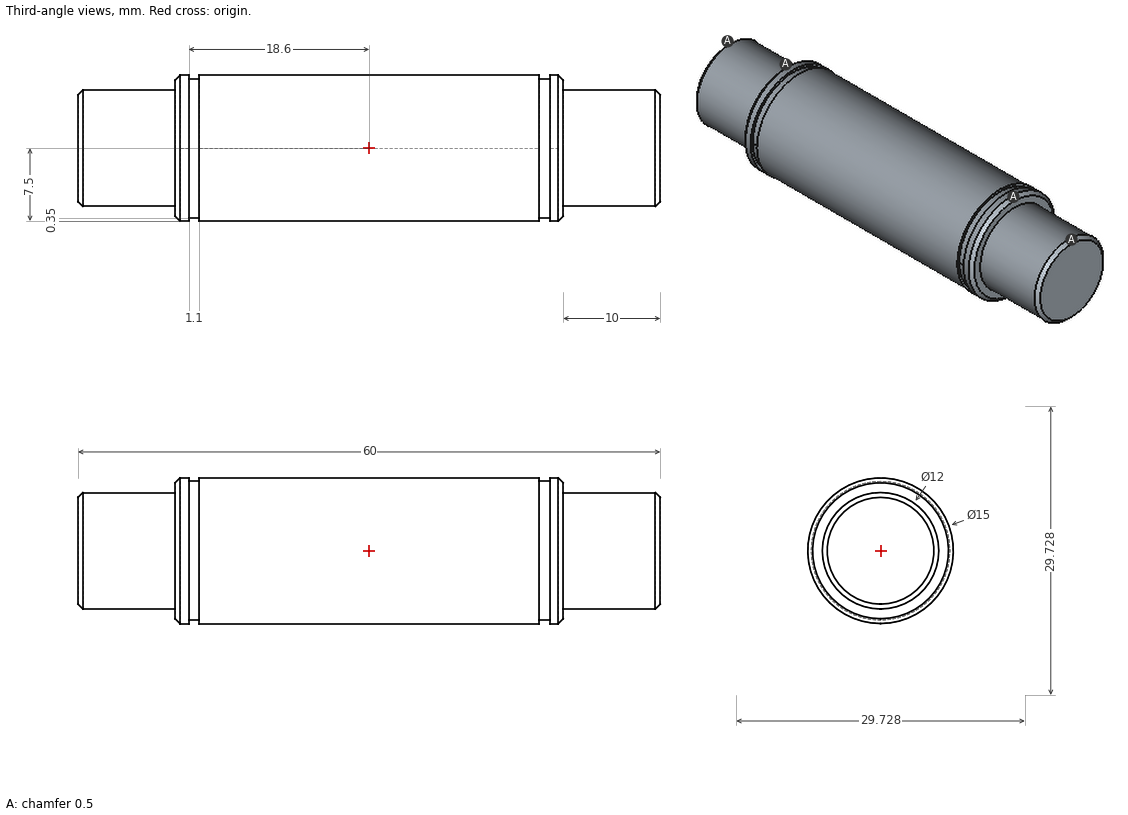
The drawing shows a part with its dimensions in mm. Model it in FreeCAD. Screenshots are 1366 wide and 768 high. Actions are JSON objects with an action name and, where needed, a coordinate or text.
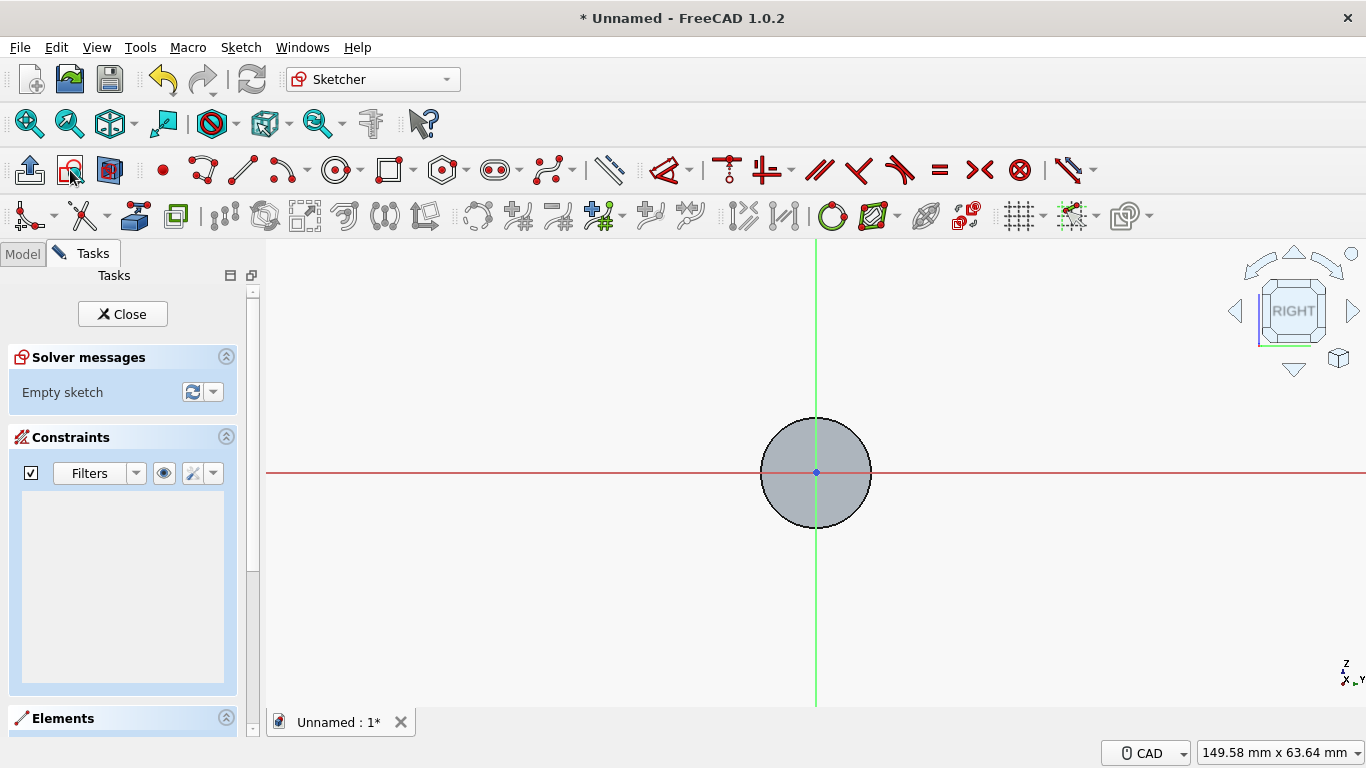
{"action": "left_click", "coordinate": [416, 170]}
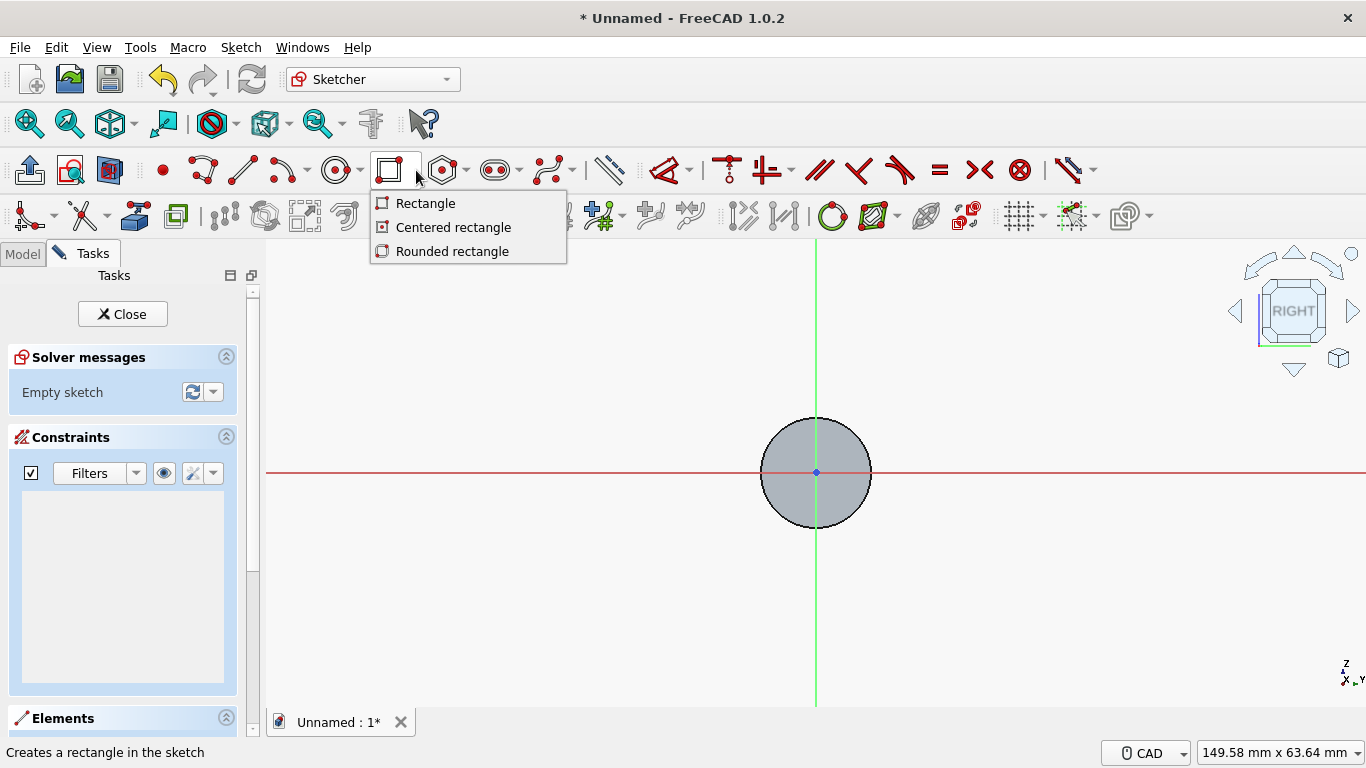
{"action": "left_click", "coordinate": [468, 227]}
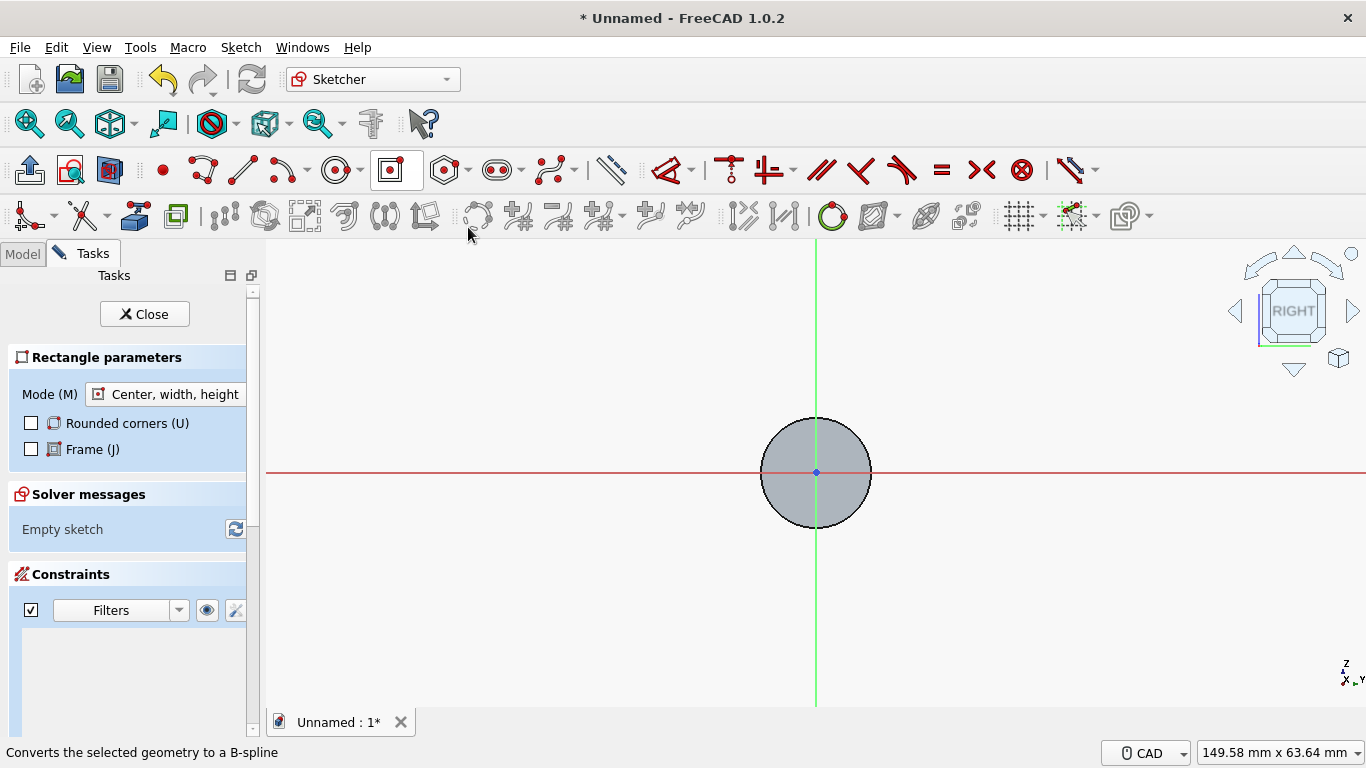
{"action": "left_click", "coordinate": [816, 473]}
{"action": "left_click", "coordinate": [925, 364]}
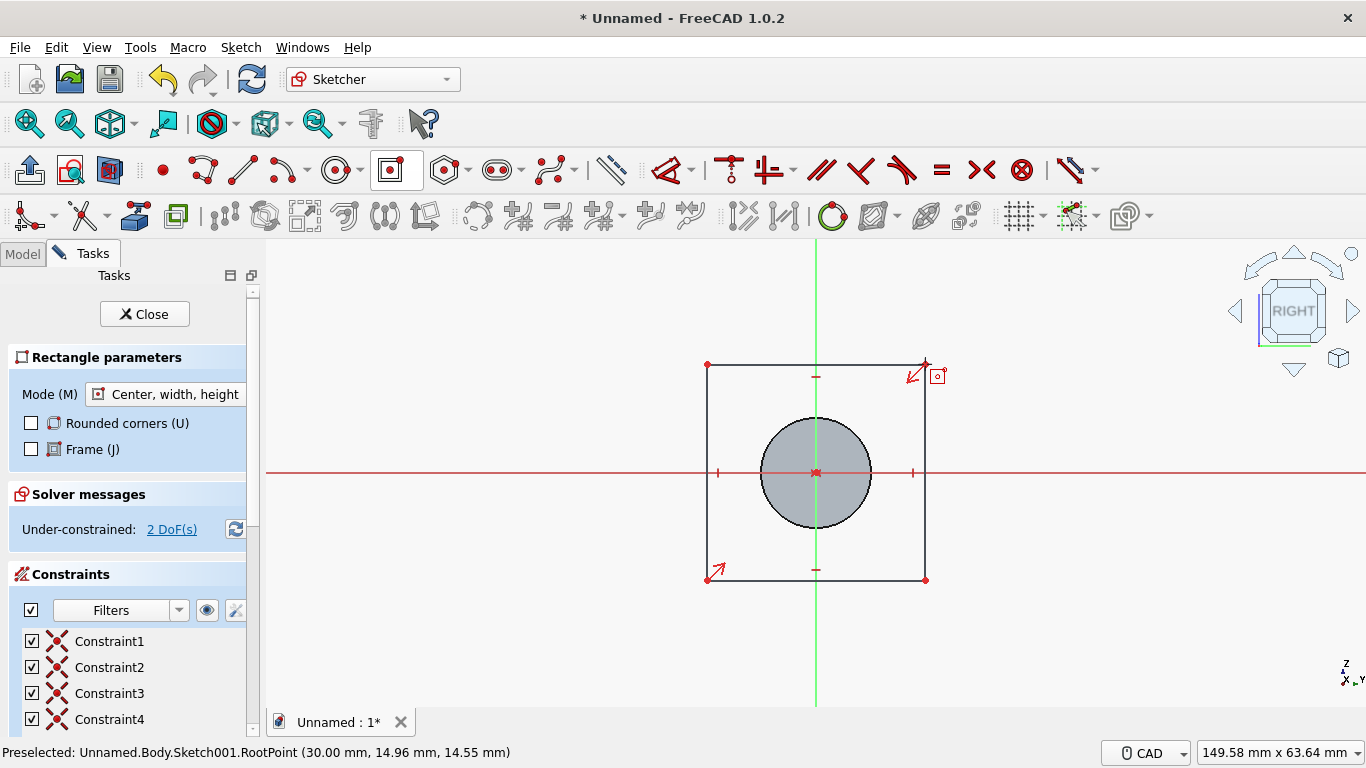
{"action": "left_click", "coordinate": [336, 170]}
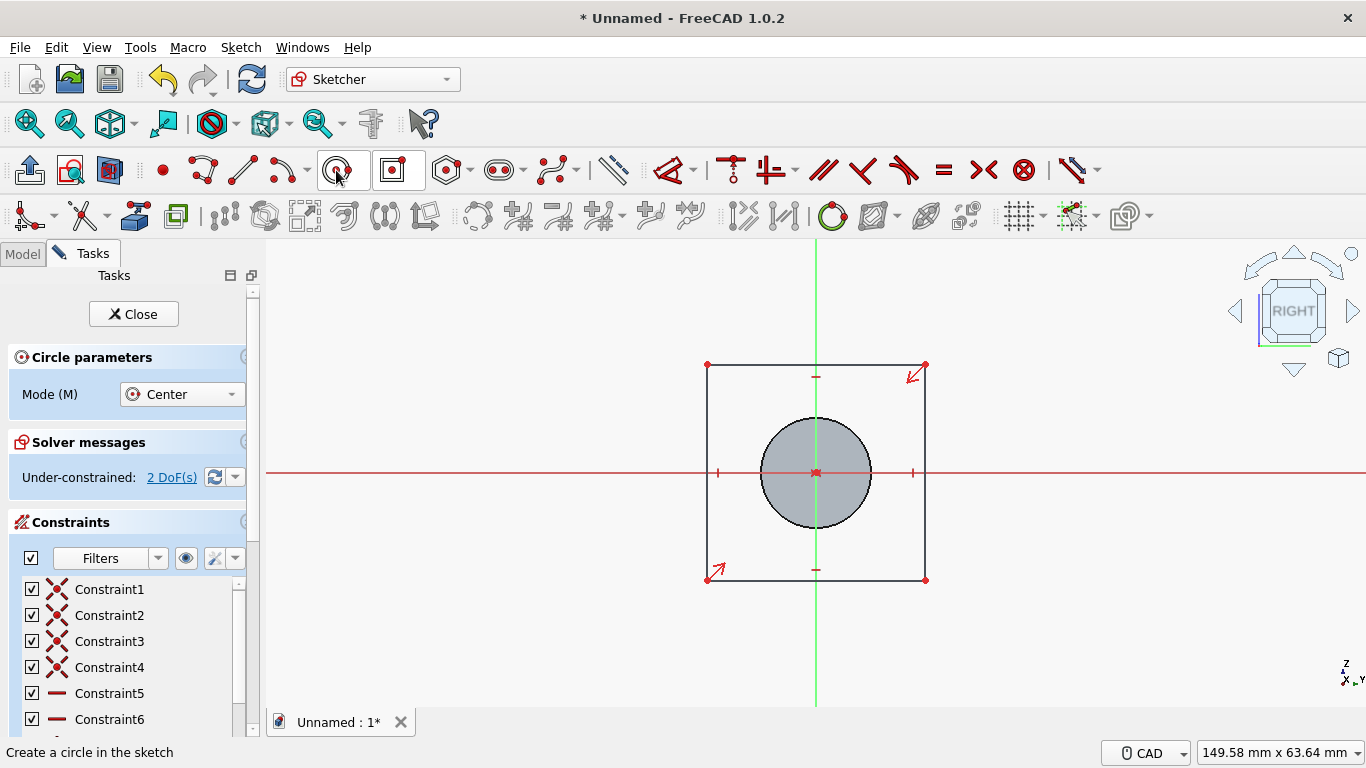
{"action": "left_click", "coordinate": [816, 473]}
{"action": "left_click", "coordinate": [847, 442]}
{"action": "key", "text": "Escape"}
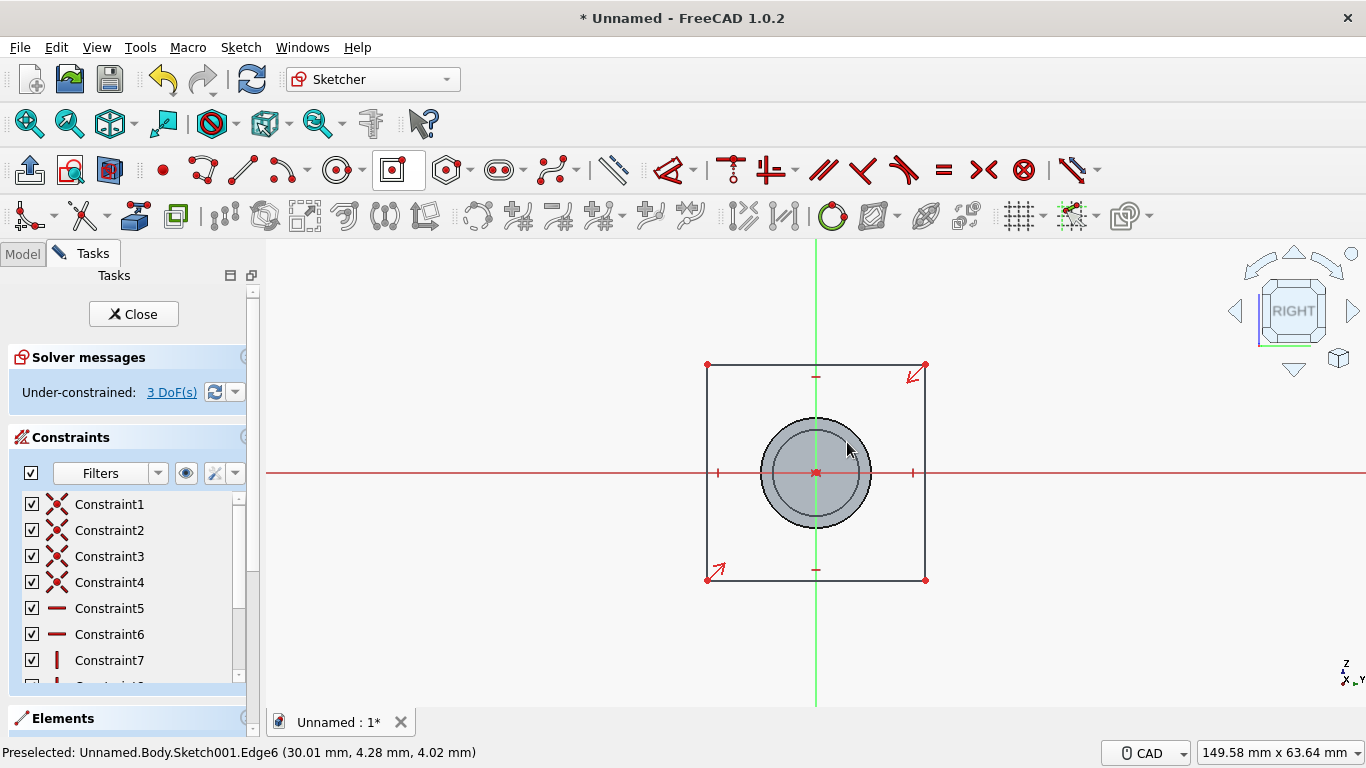
{"action": "key", "text": "d"}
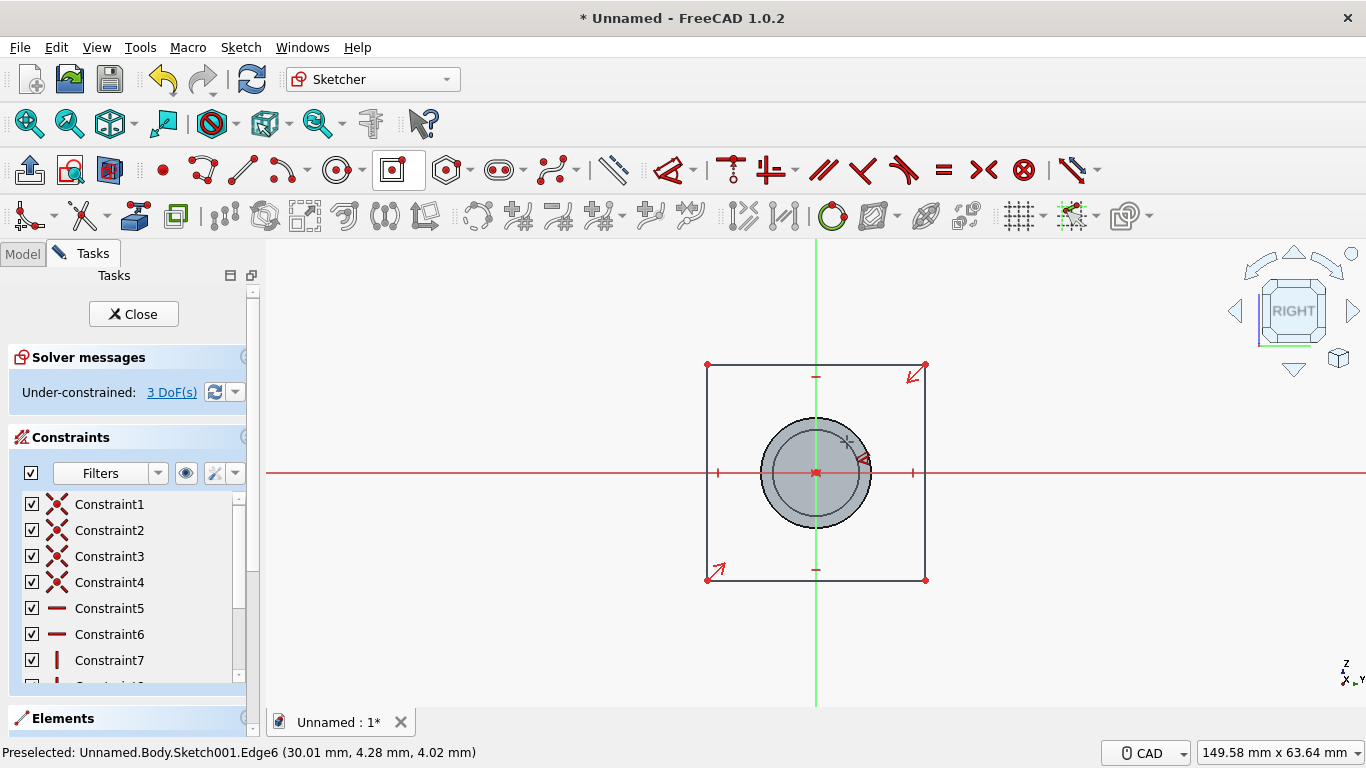
{"action": "left_click", "coordinate": [846, 442]}
{"action": "left_click", "coordinate": [868, 419]}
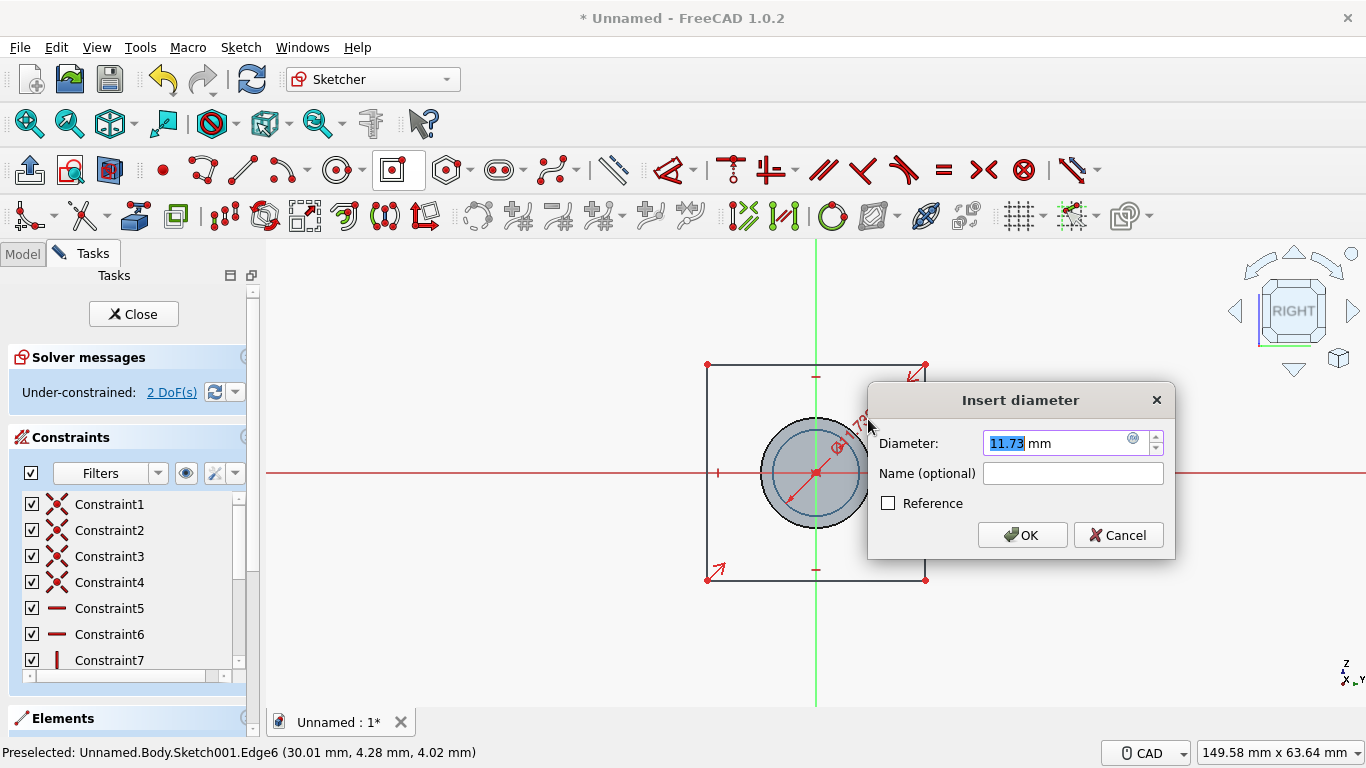
{"action": "type", "text": "12"}
{"action": "key", "text": "Return"}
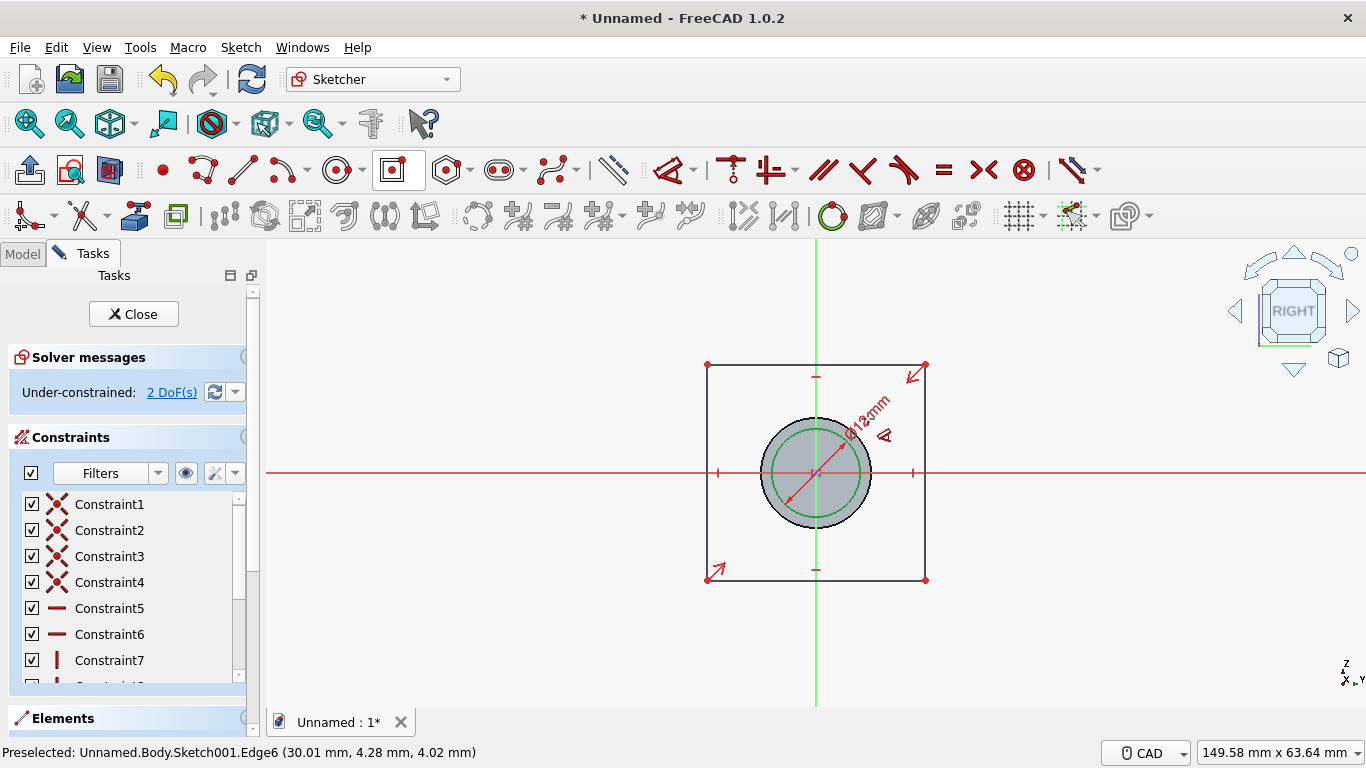
{"action": "left_click", "coordinate": [772, 581]}
{"action": "left_click", "coordinate": [766, 615]}